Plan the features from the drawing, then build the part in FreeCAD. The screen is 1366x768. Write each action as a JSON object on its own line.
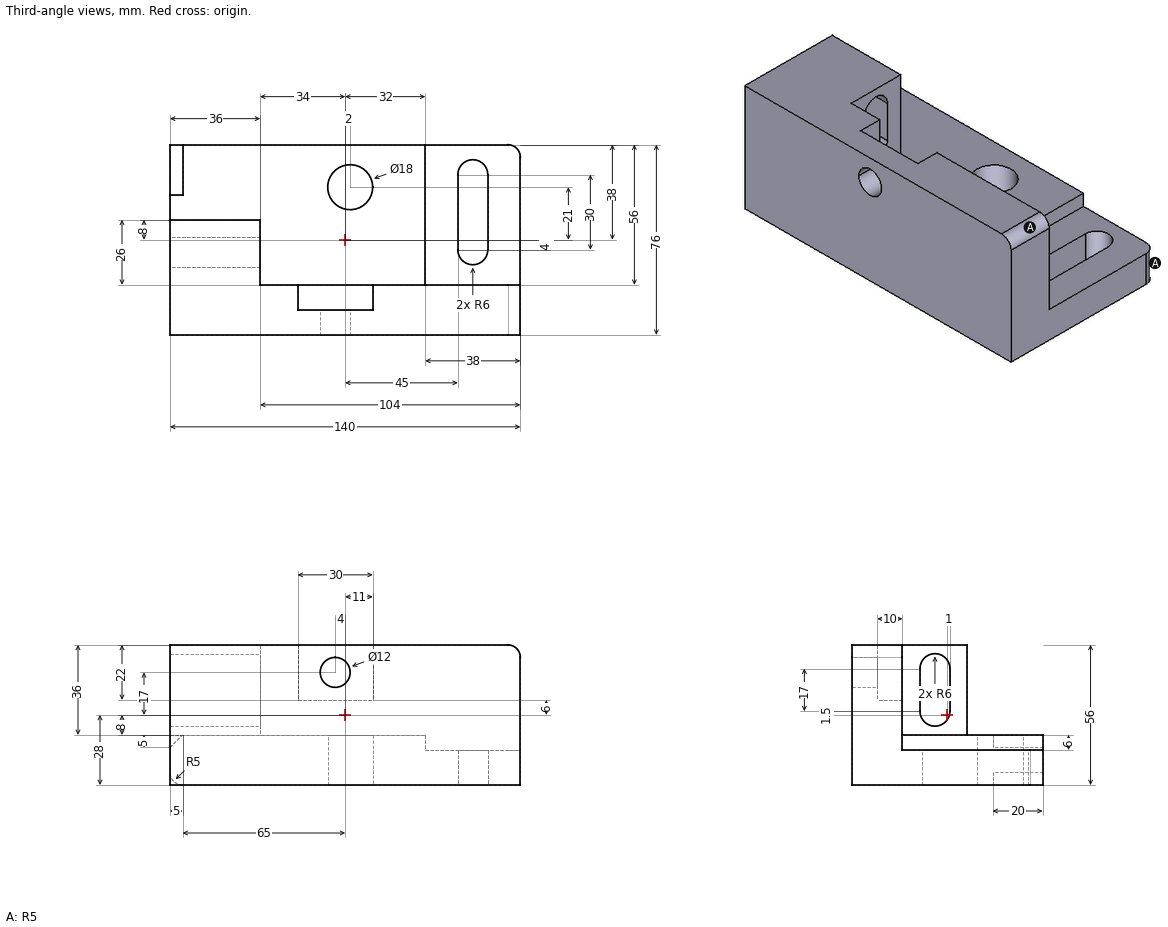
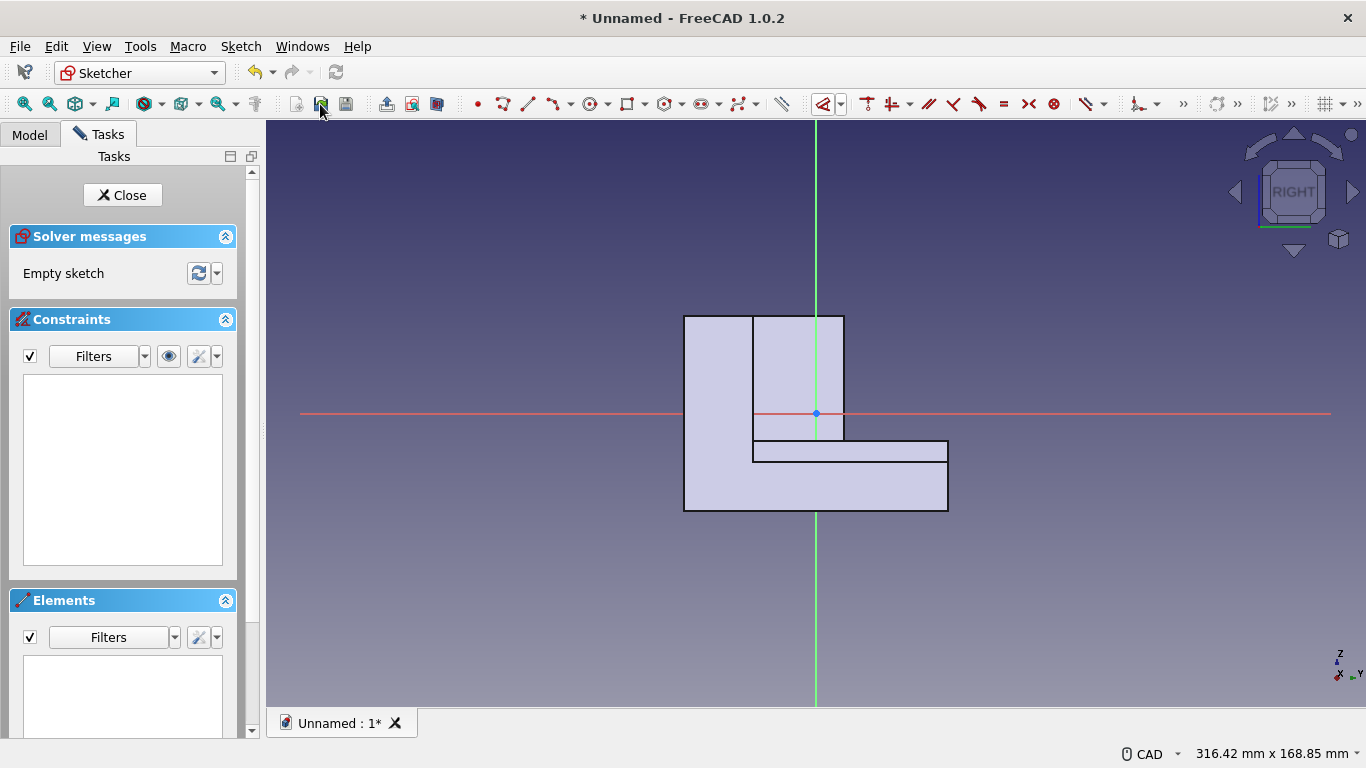
{"action": "scroll", "coordinate": [815, 367], "scroll_direction": "up", "scroll_amount": 7}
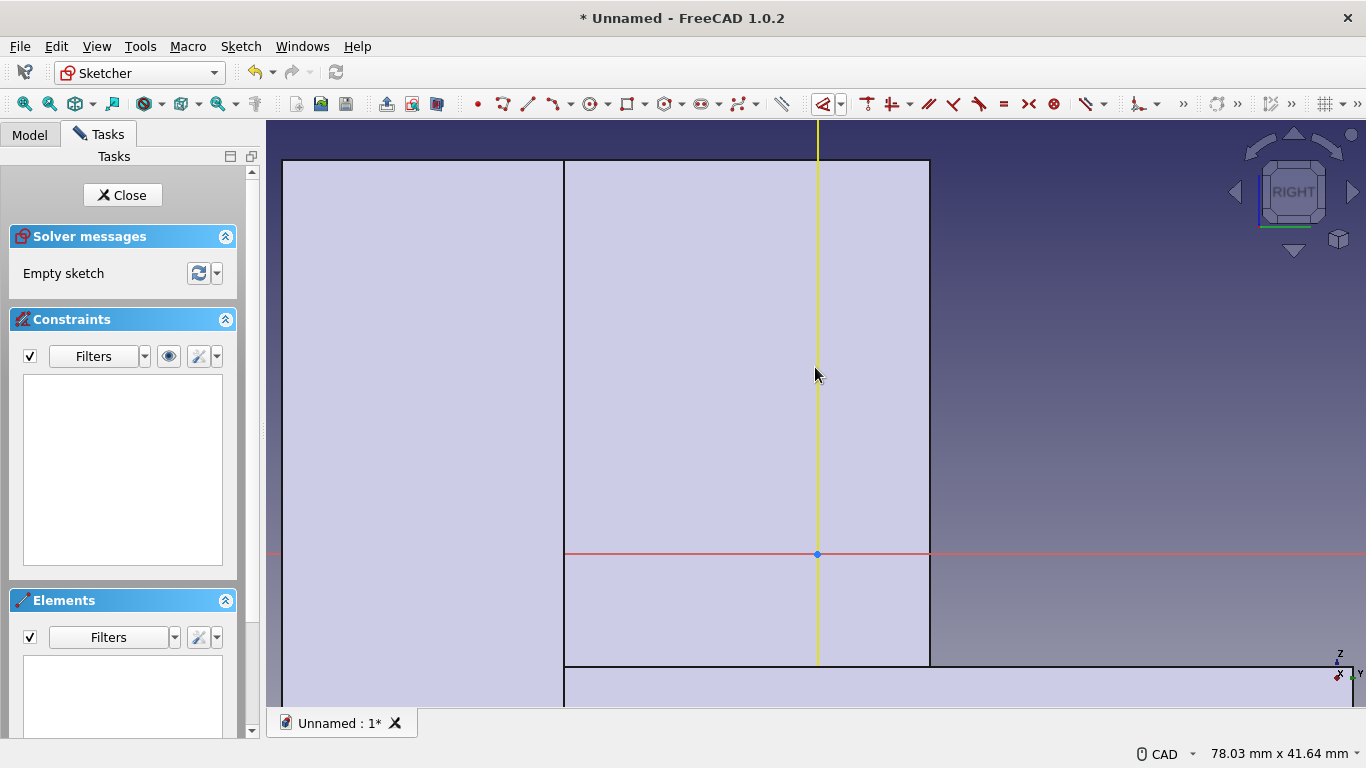
{"action": "key", "text": "g s"}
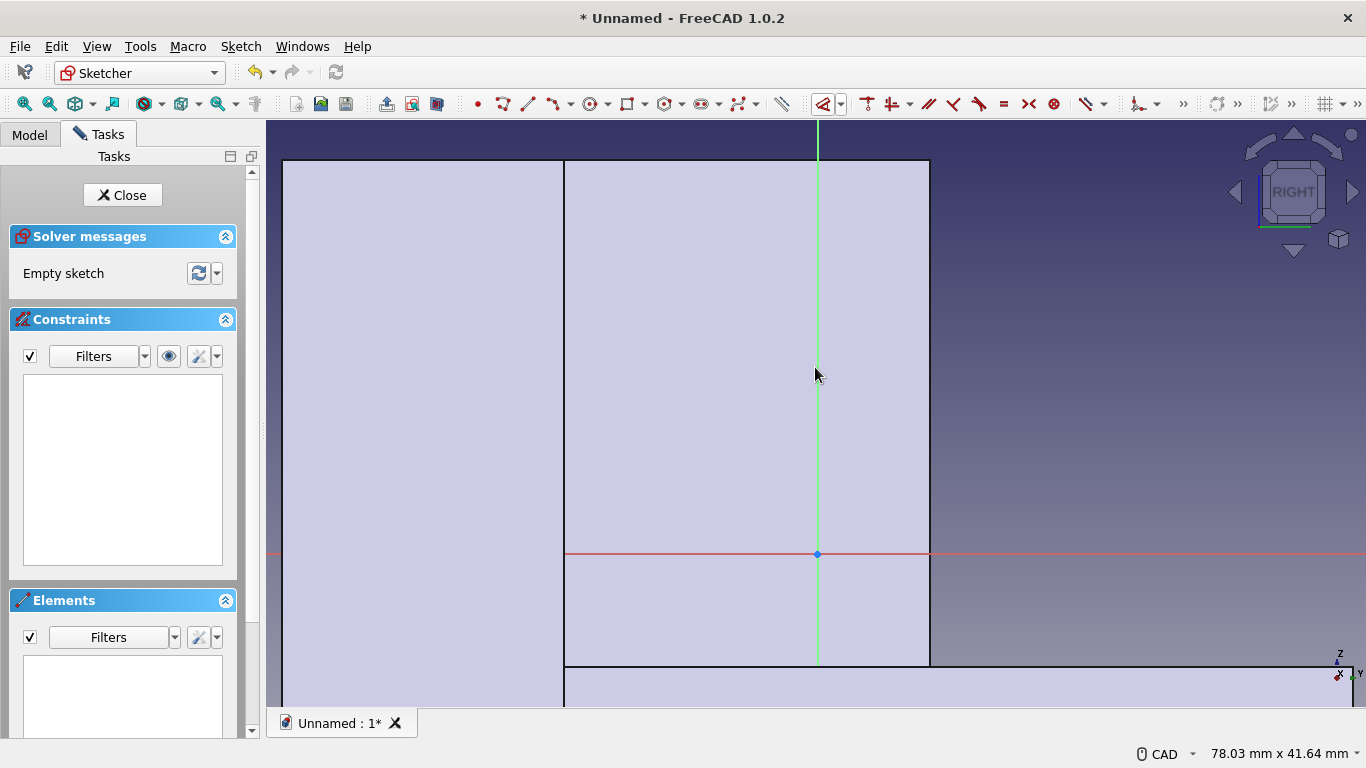
{"action": "left_click", "coordinate": [747, 533]}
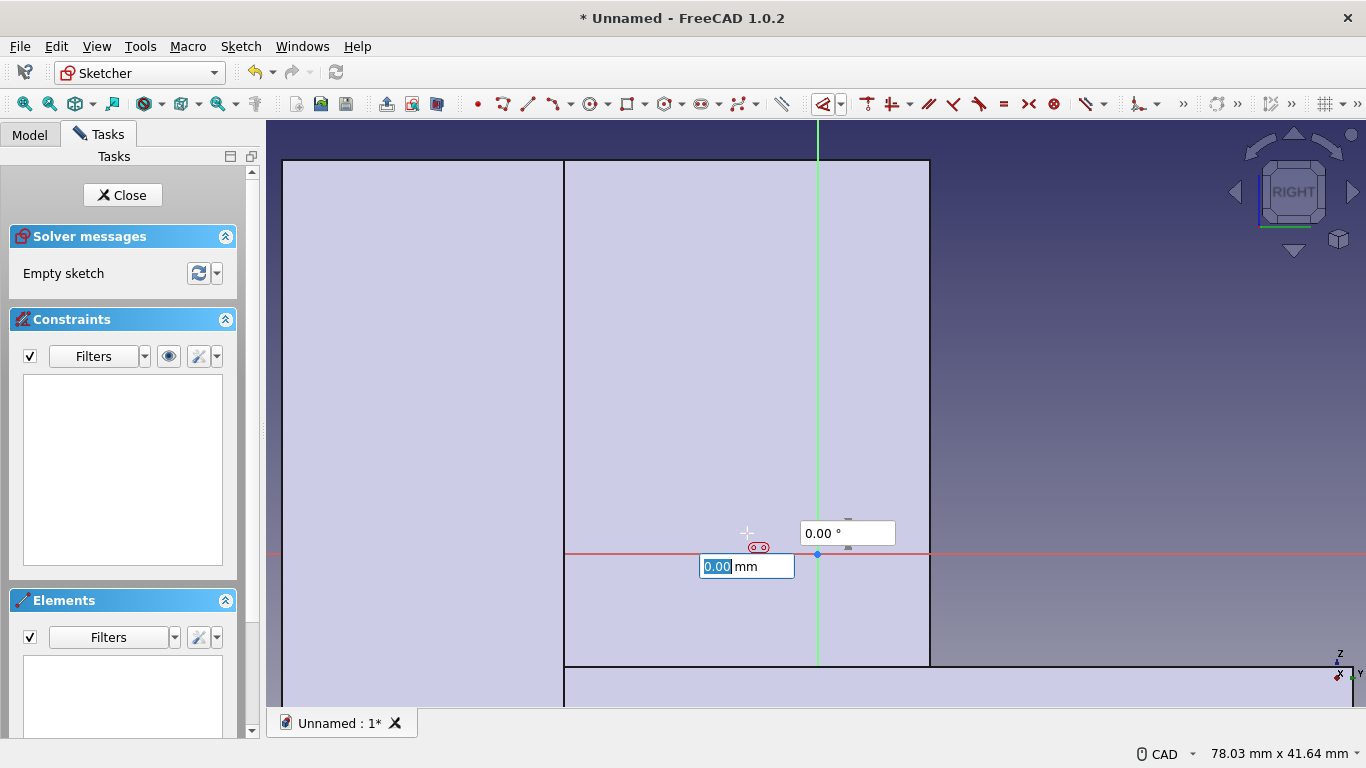
{"action": "left_click", "coordinate": [747, 293]}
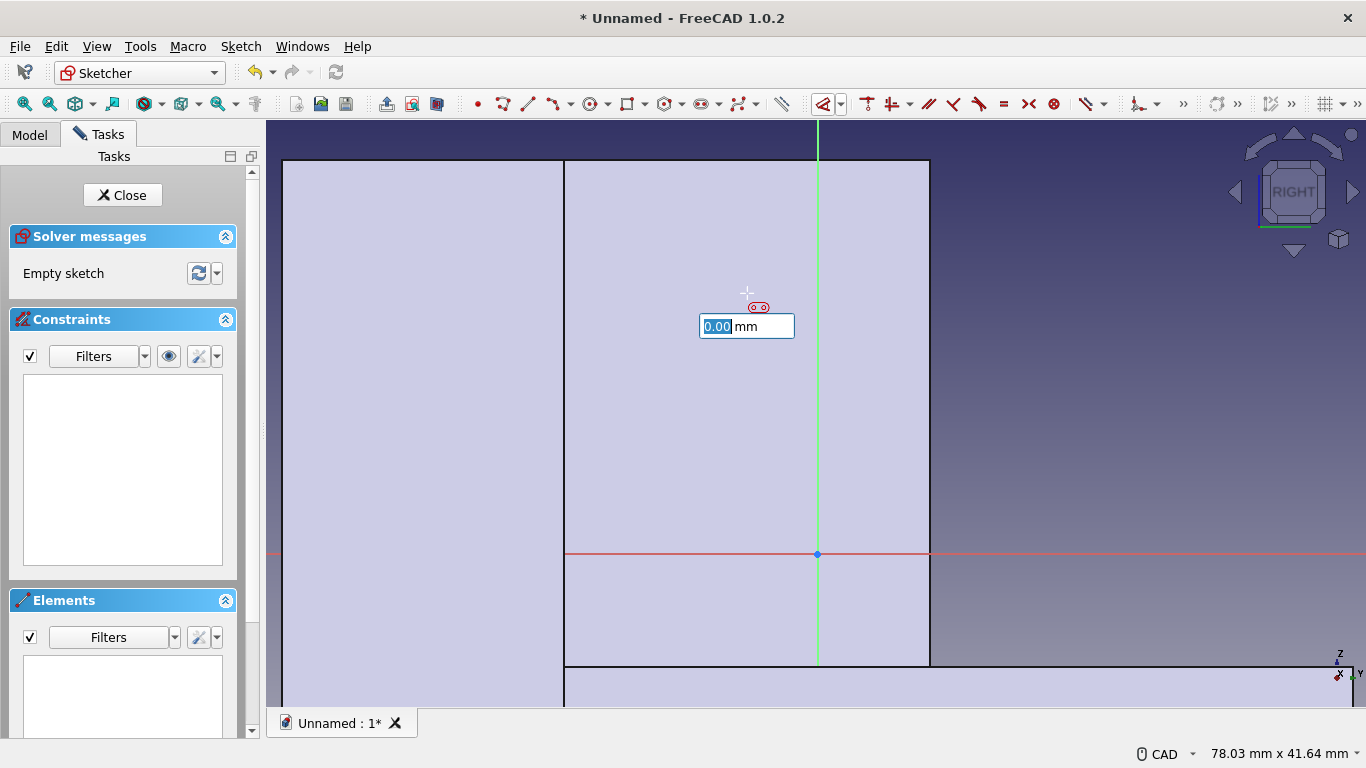
{"action": "left_click", "coordinate": [832, 413]}
{"action": "key", "text": "Escape"}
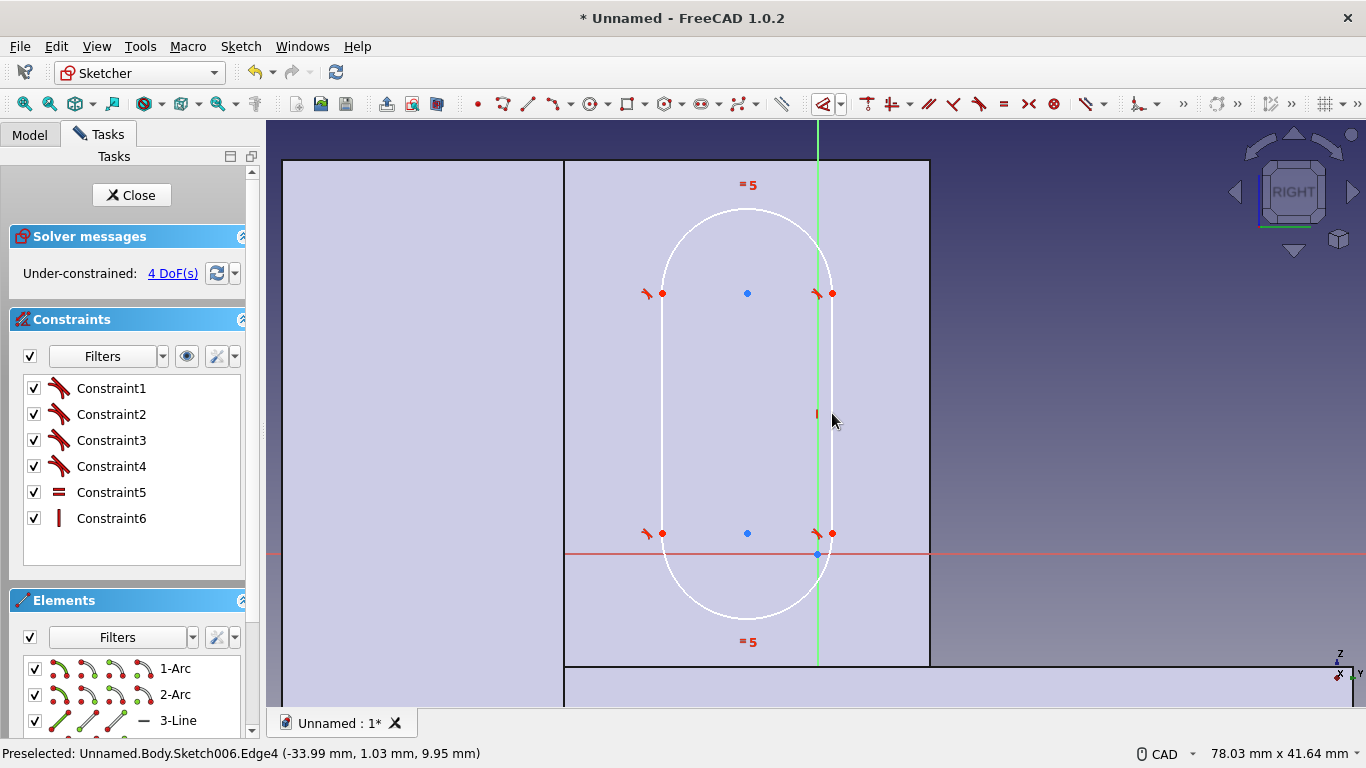
{"action": "left_click", "coordinate": [697, 603]}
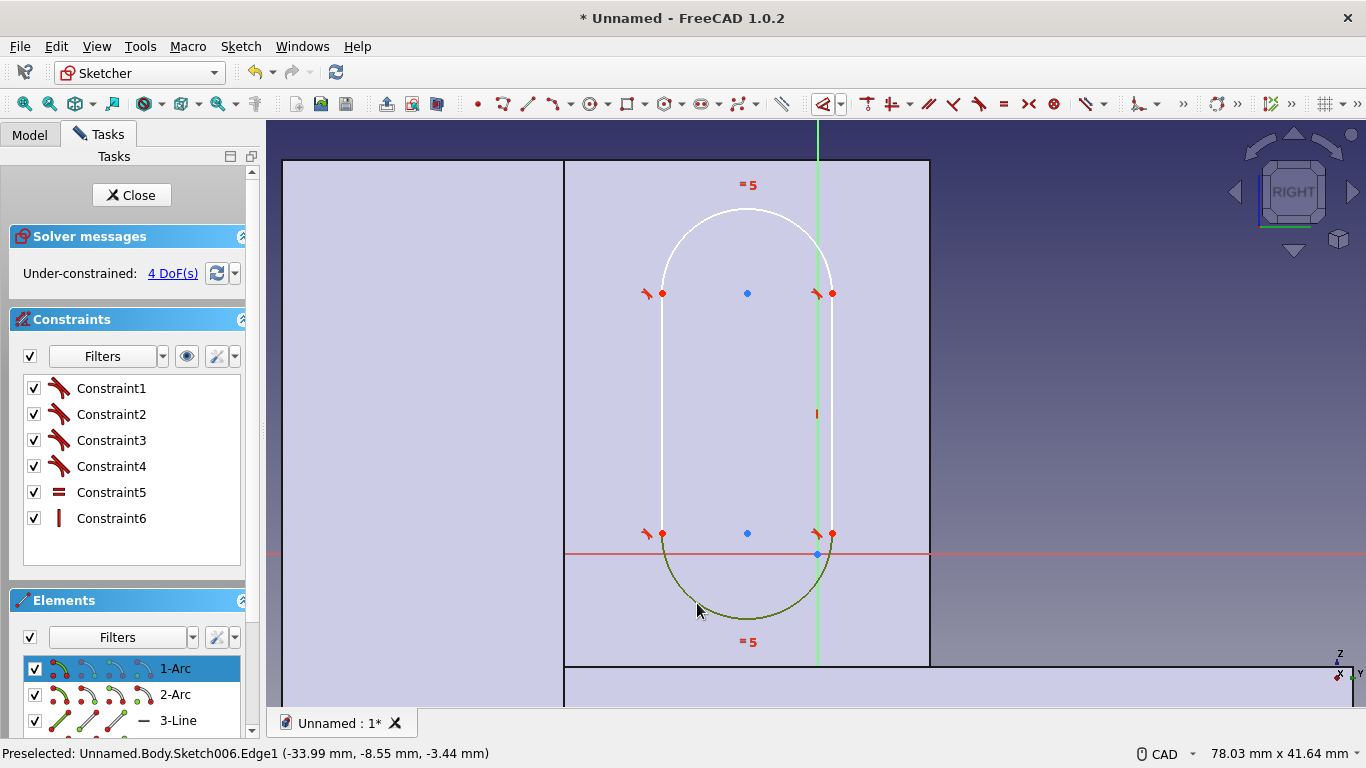
{"action": "left_click", "coordinate": [840, 104]}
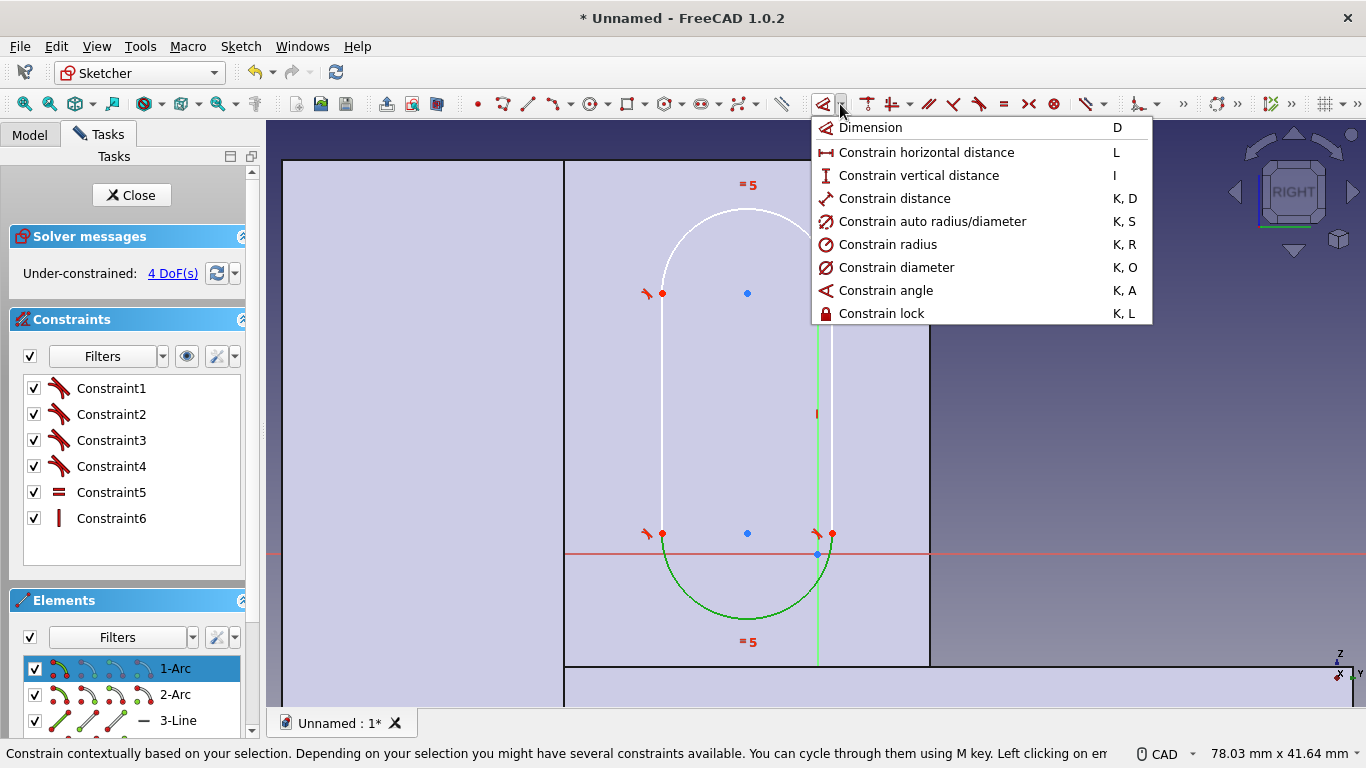
{"action": "left_click", "coordinate": [982, 244]}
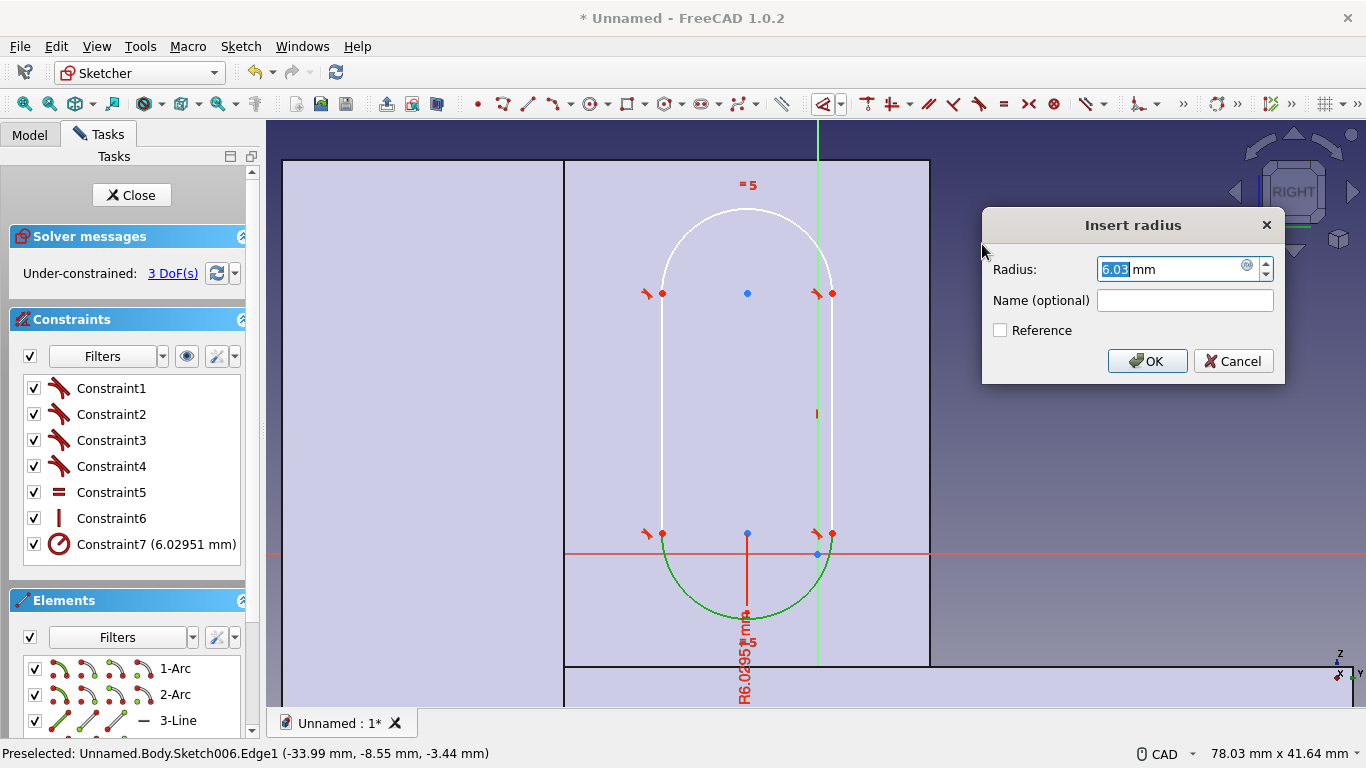
{"action": "type", "text": "6"}
{"action": "key", "text": "Return"}